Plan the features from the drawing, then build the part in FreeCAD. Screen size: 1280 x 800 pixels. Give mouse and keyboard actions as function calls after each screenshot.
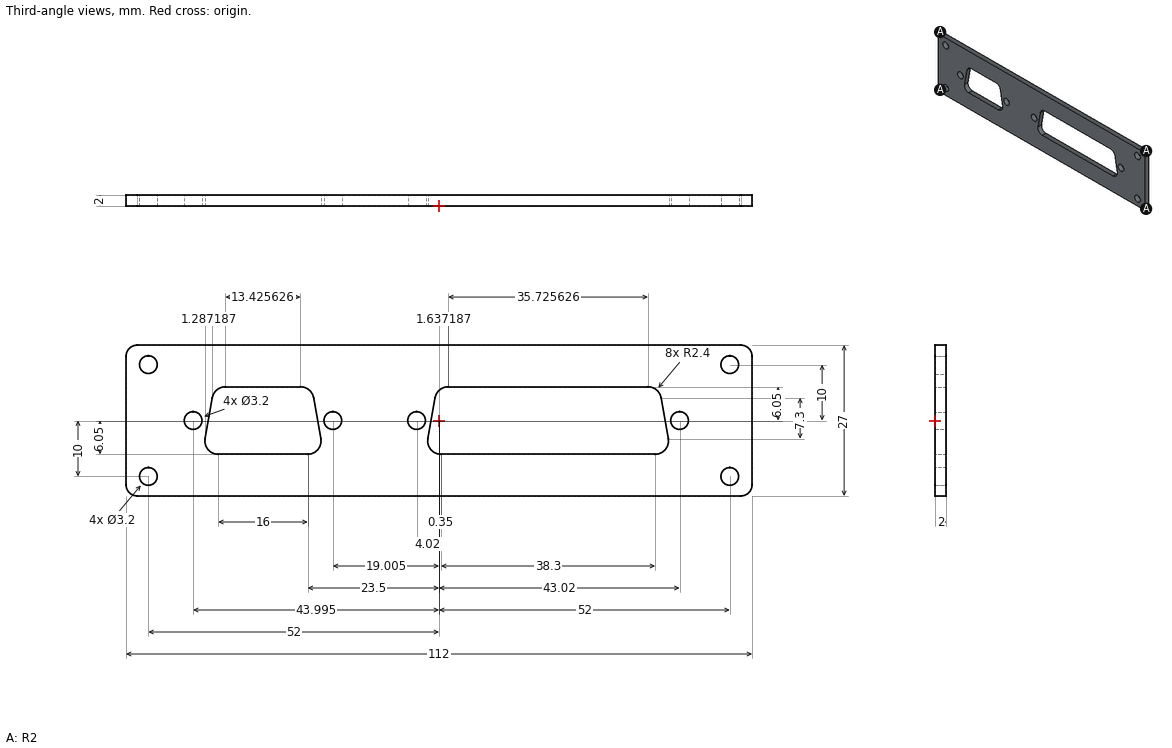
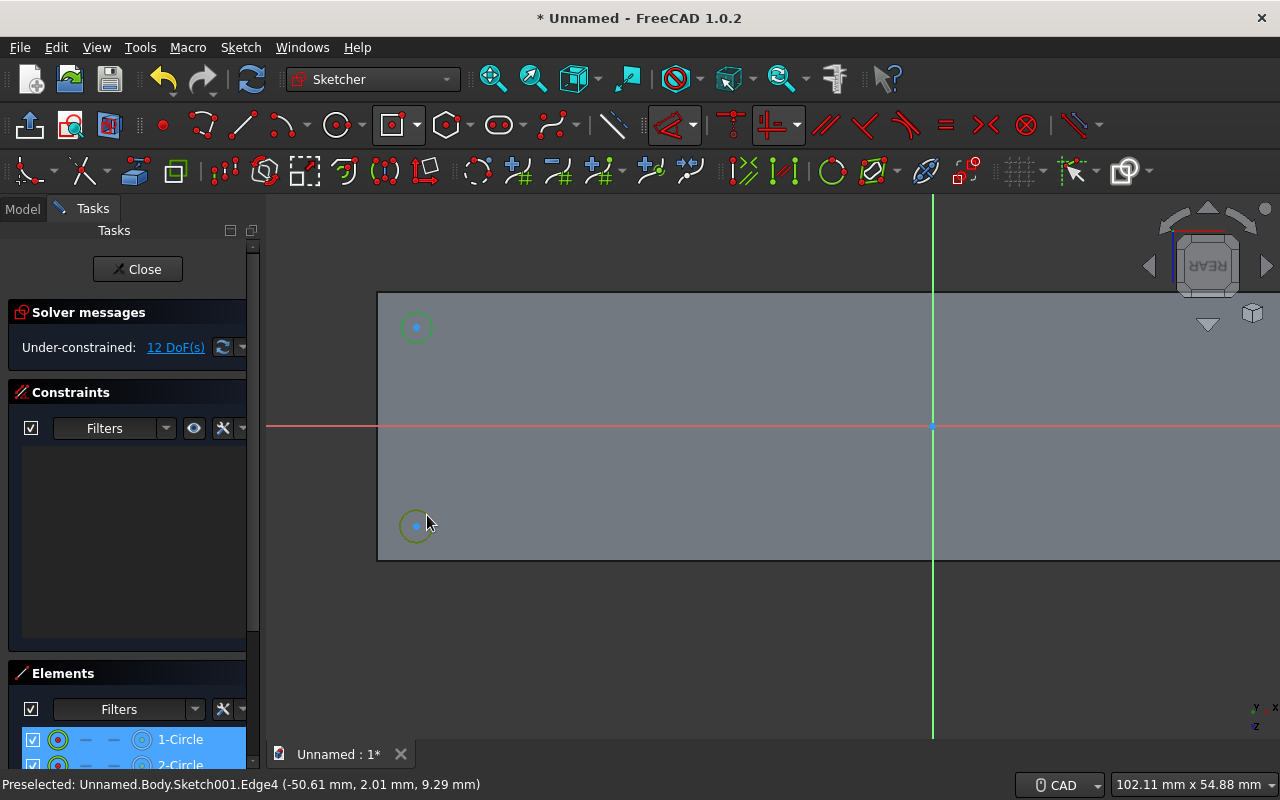
key(e)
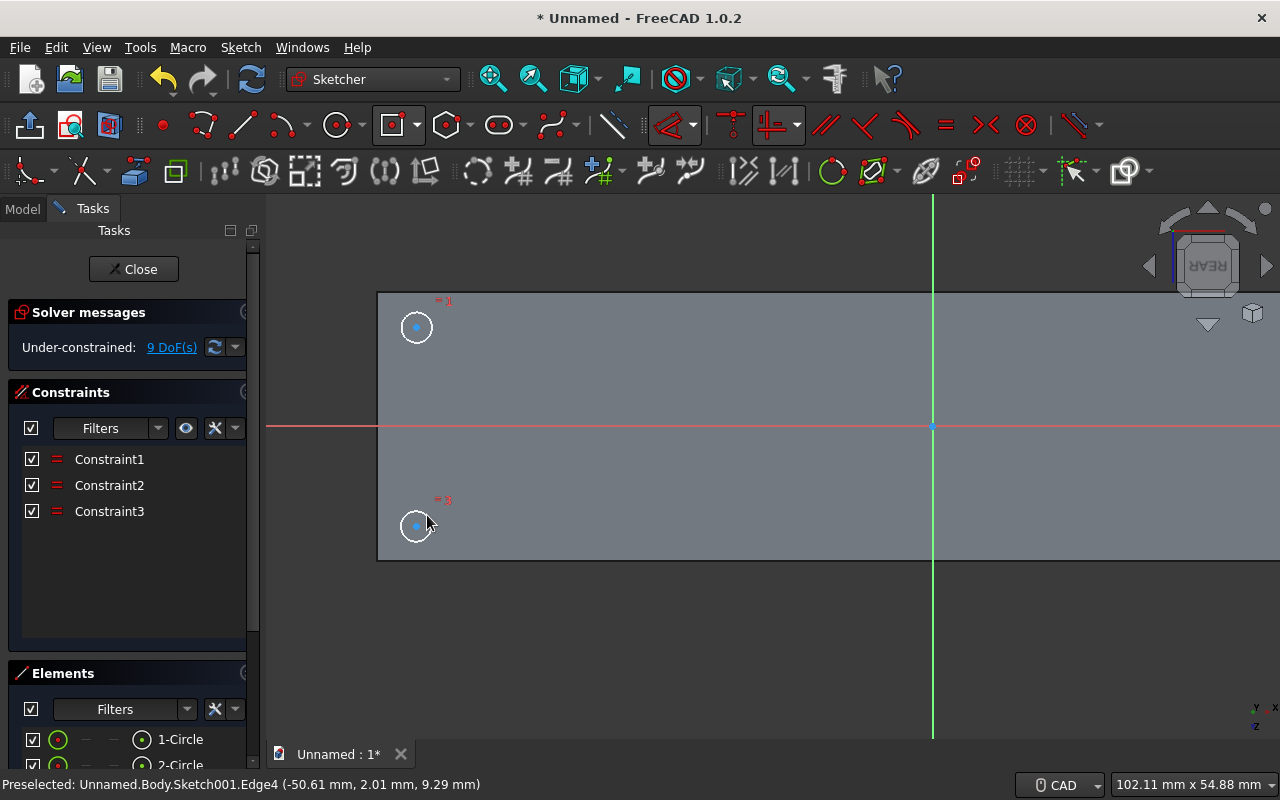
click(417, 328)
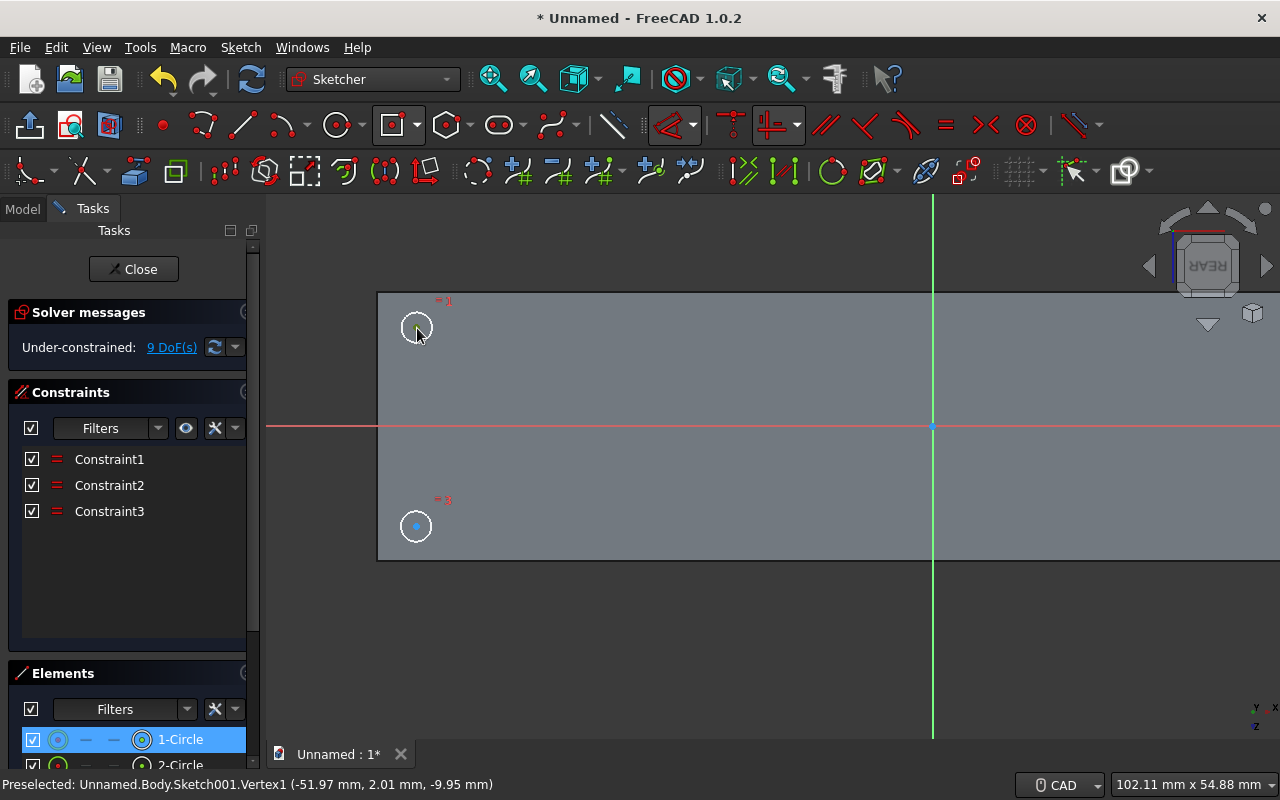
scroll(427, 515, down, 3)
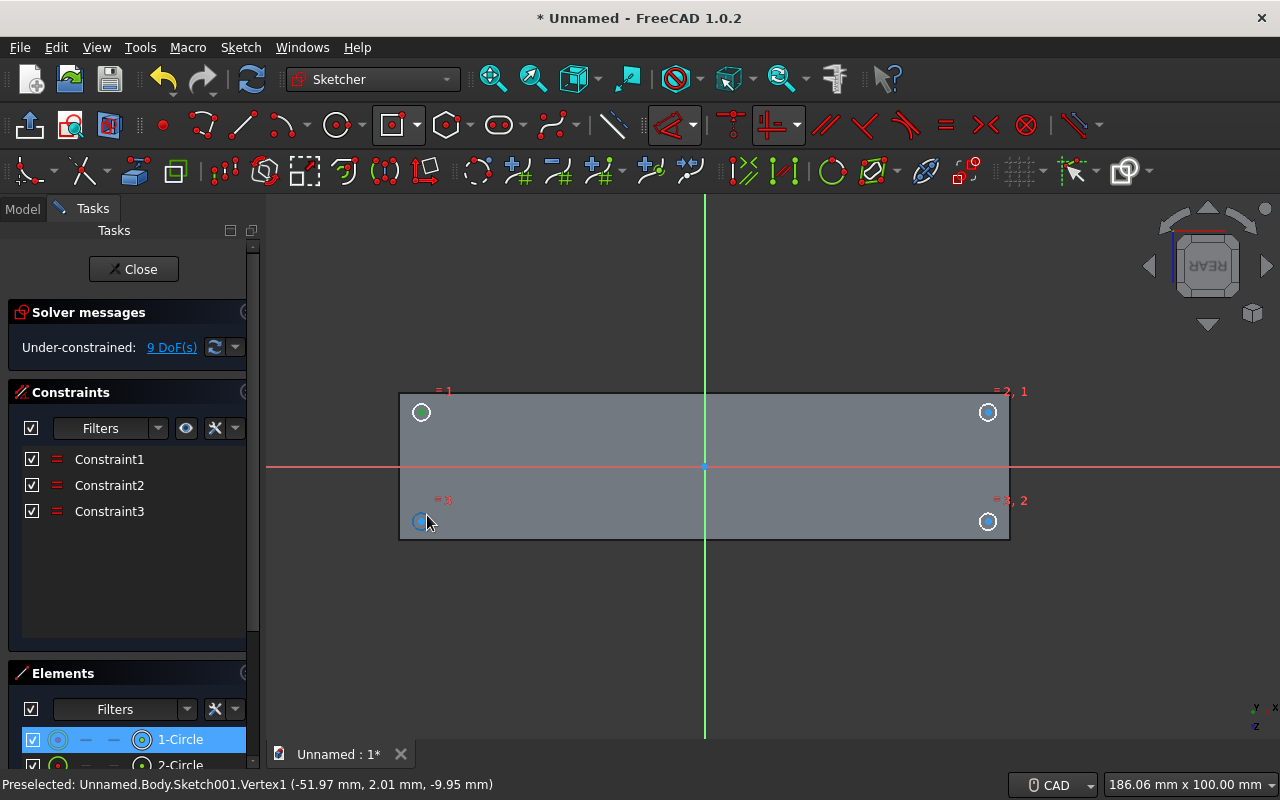
click(988, 412)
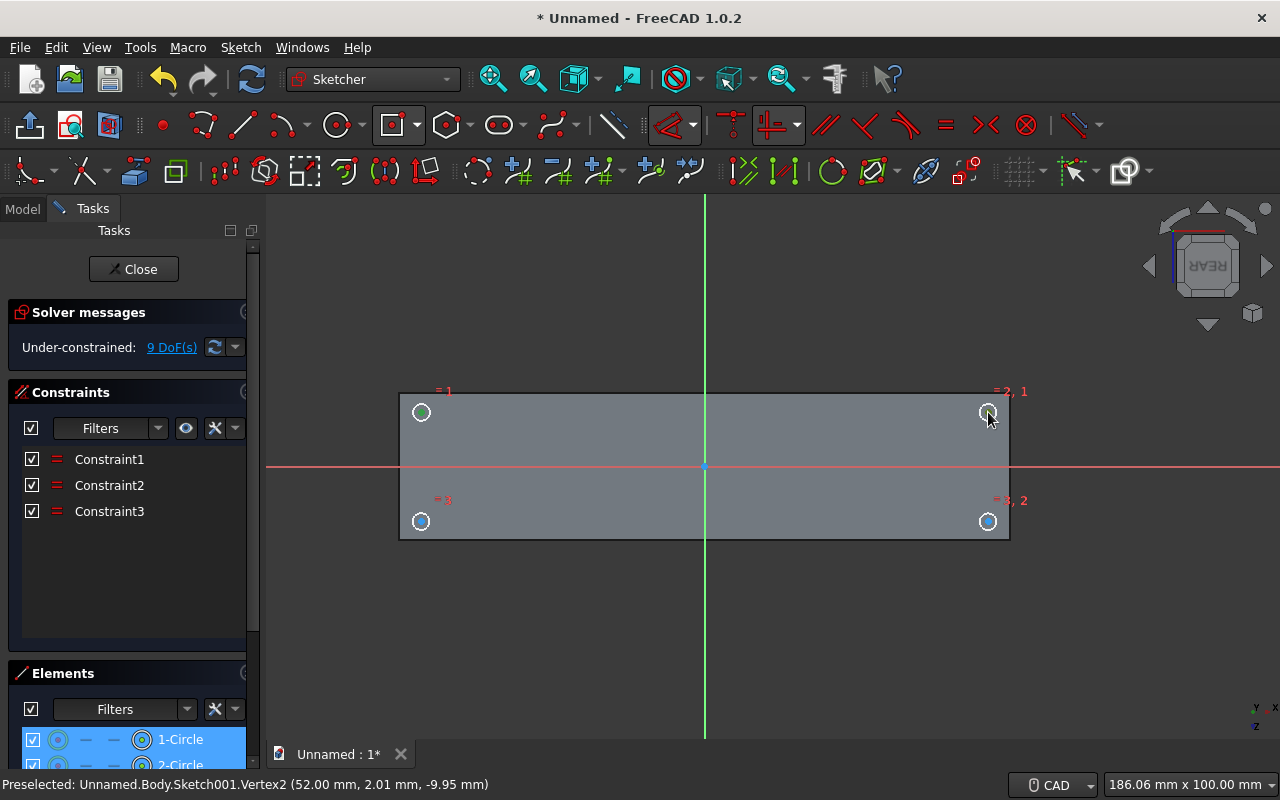
key(h)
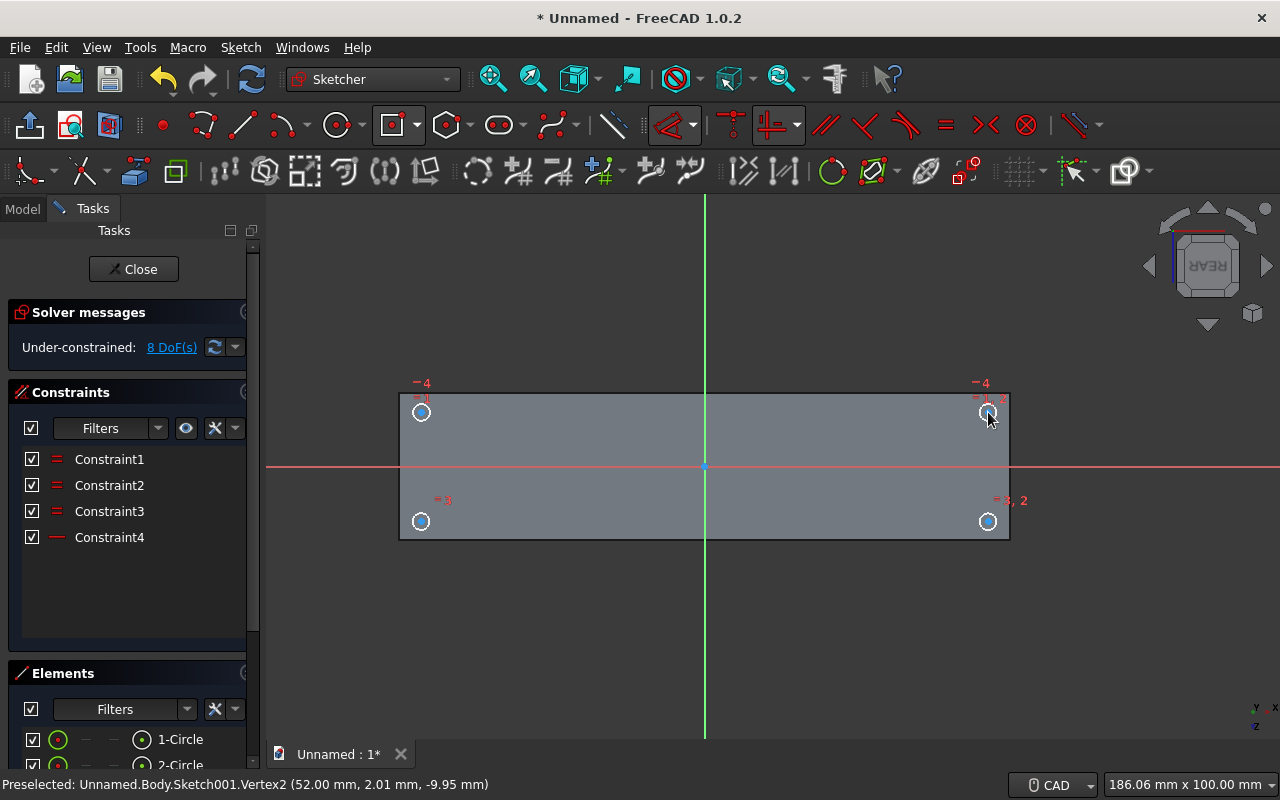
click(988, 412)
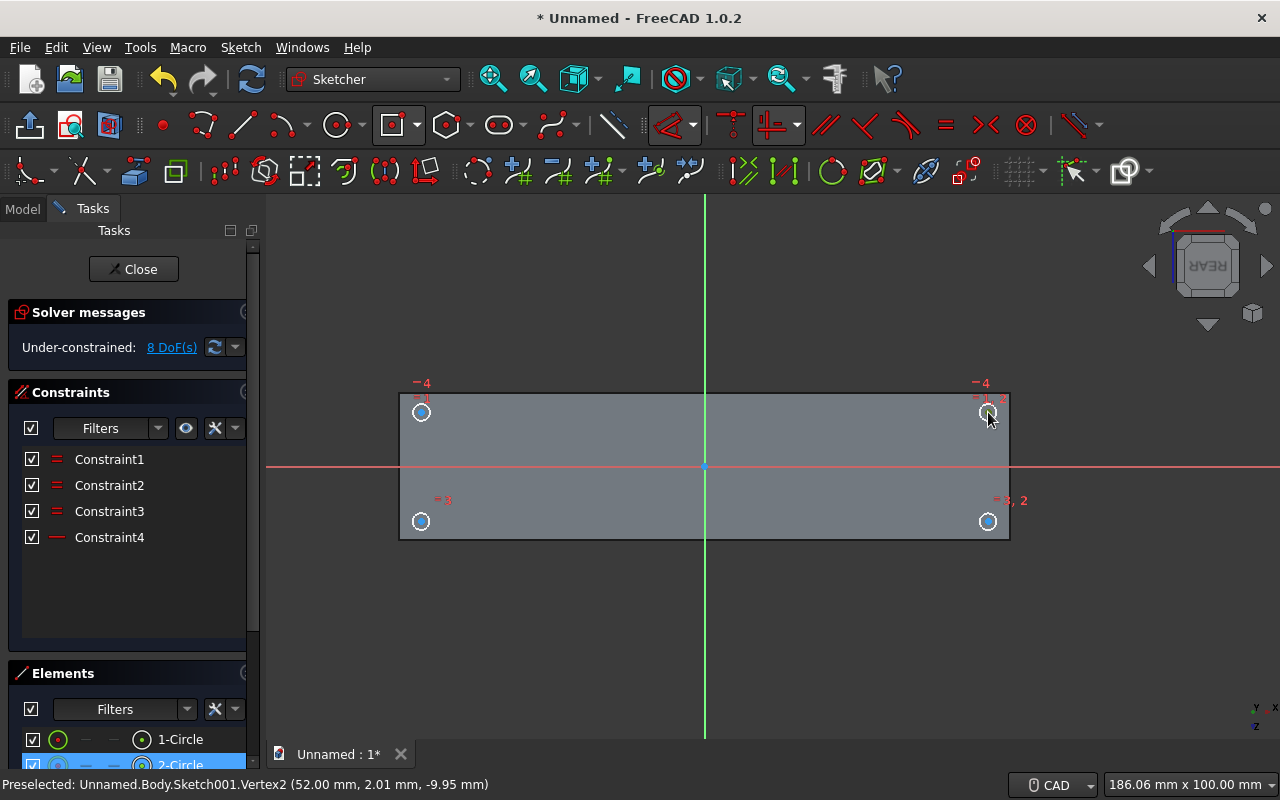
click(988, 522)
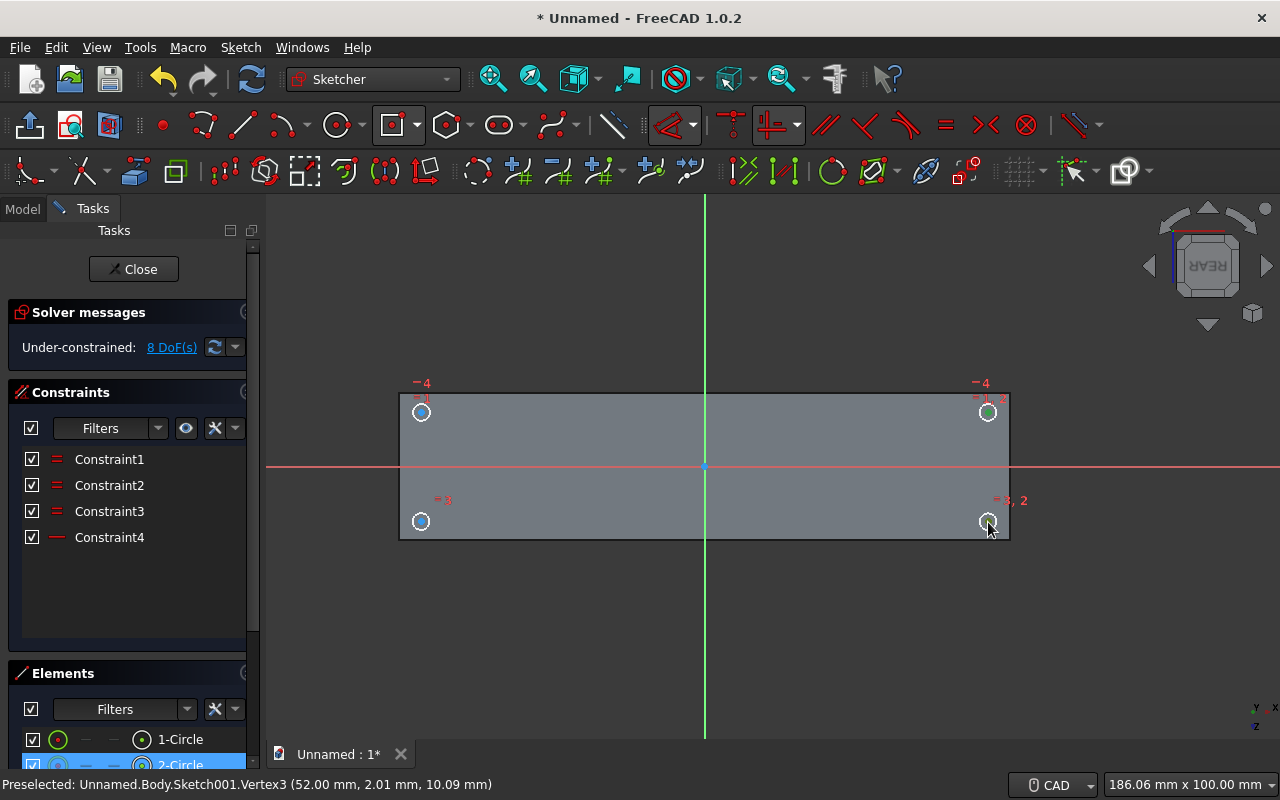
click(800, 126)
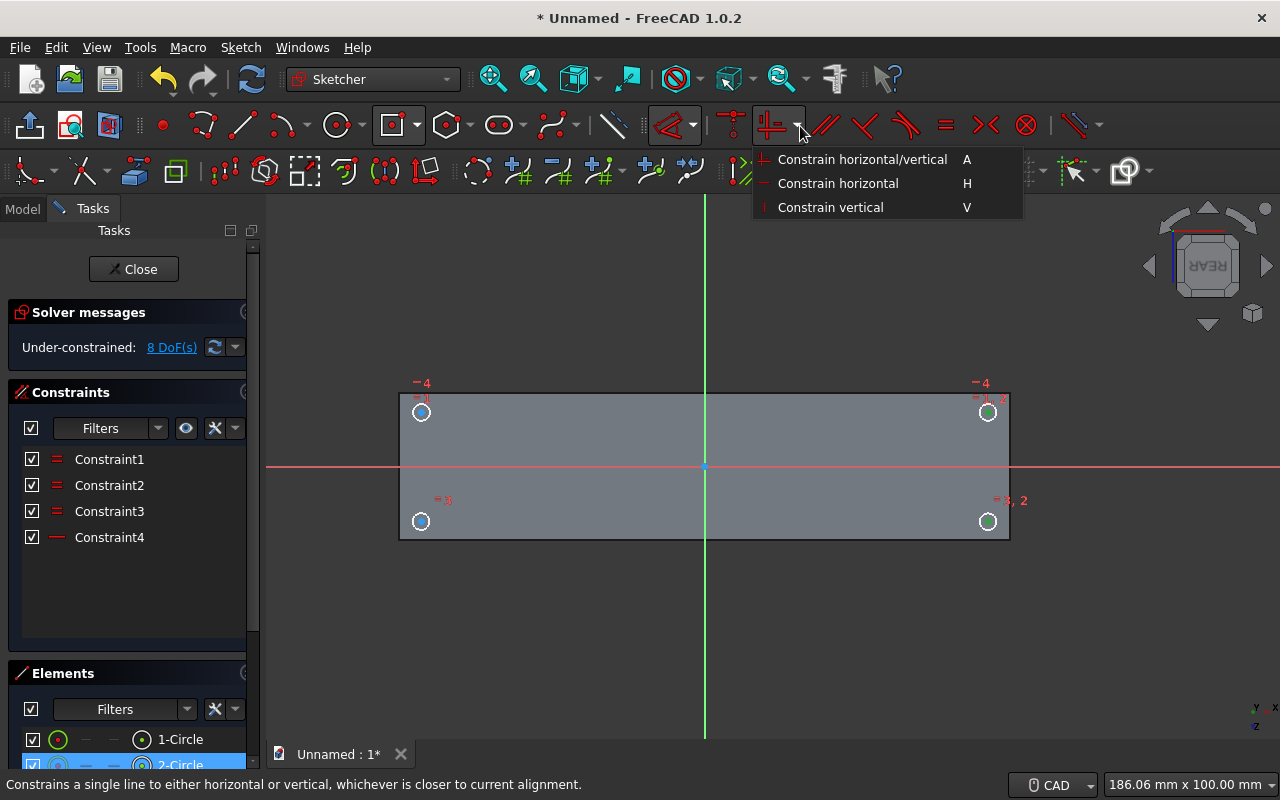
click(888, 207)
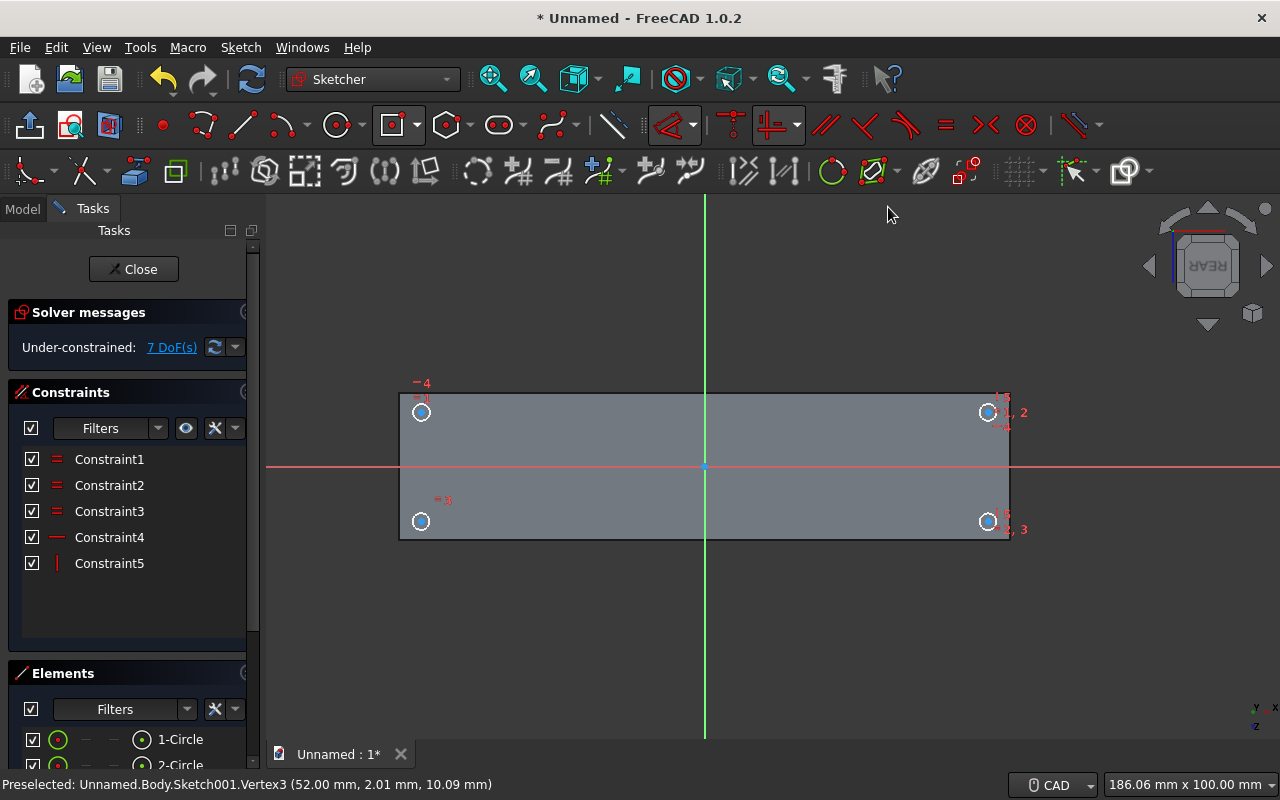
click(421, 412)